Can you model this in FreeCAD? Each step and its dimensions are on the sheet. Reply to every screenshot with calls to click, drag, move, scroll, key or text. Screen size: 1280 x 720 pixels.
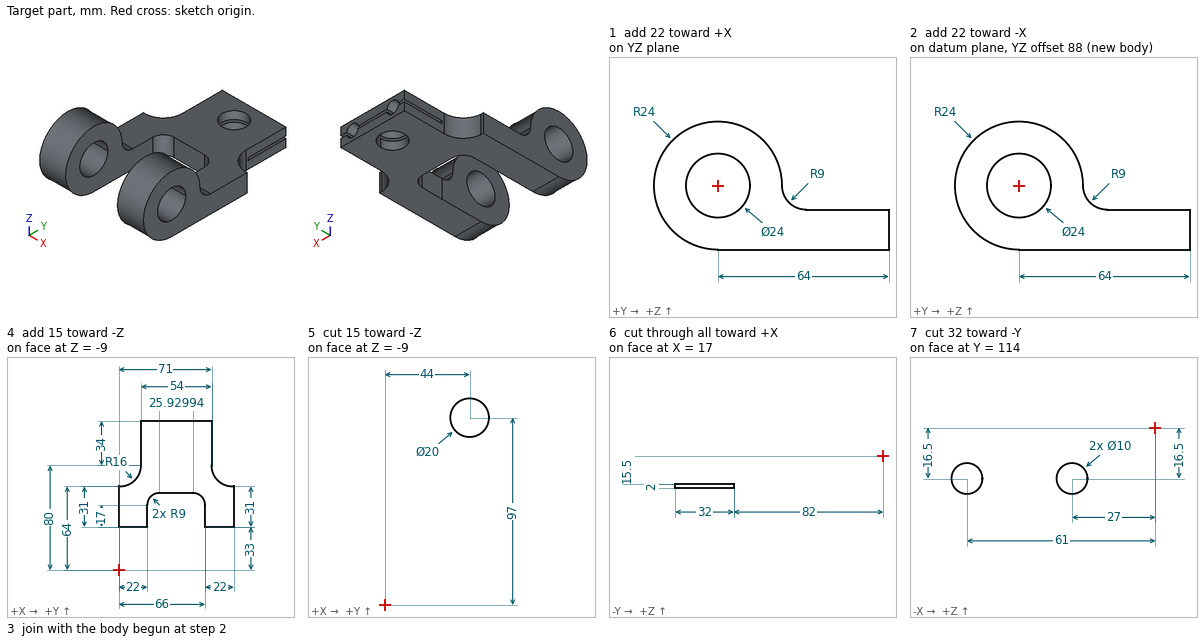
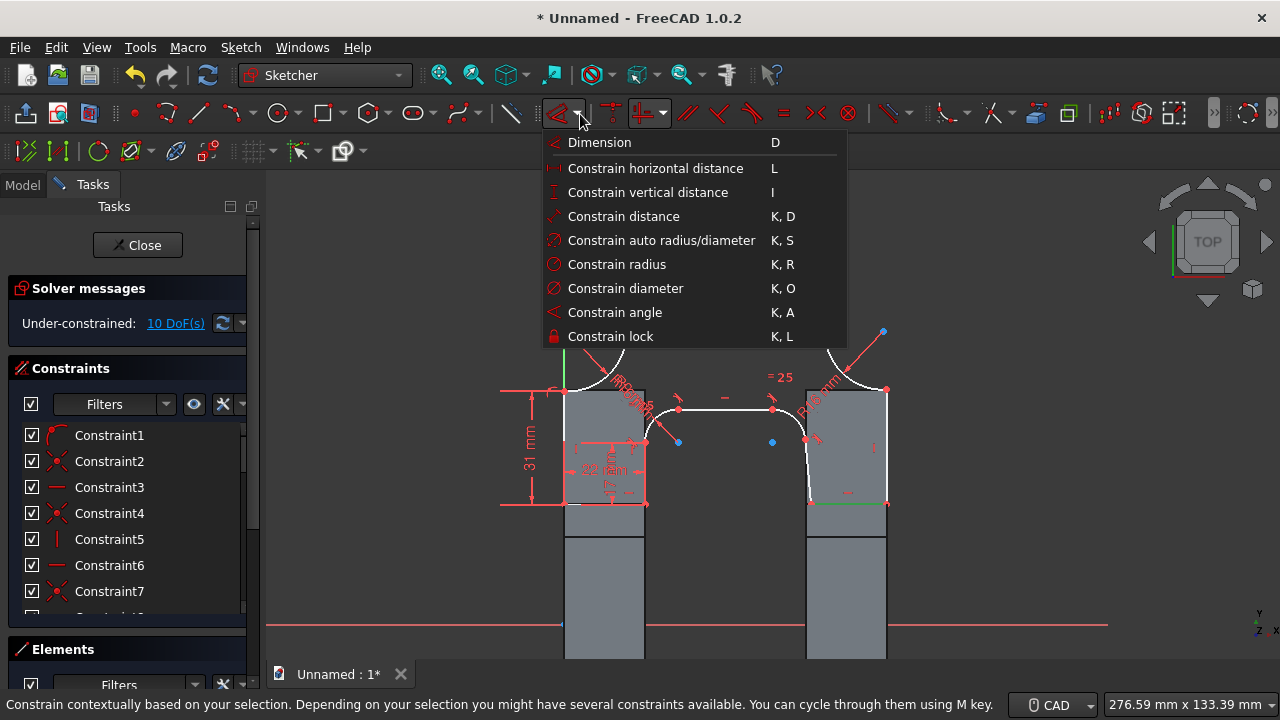
click(695, 168)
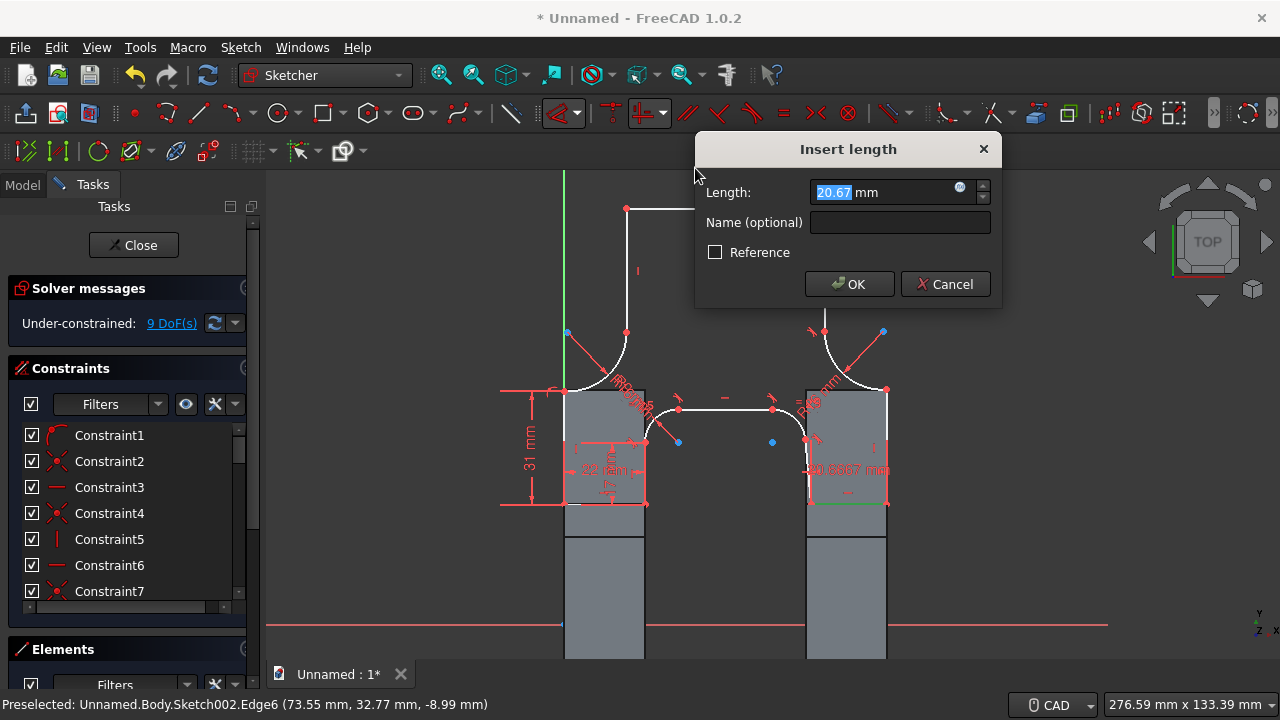
text(22)
key(Return)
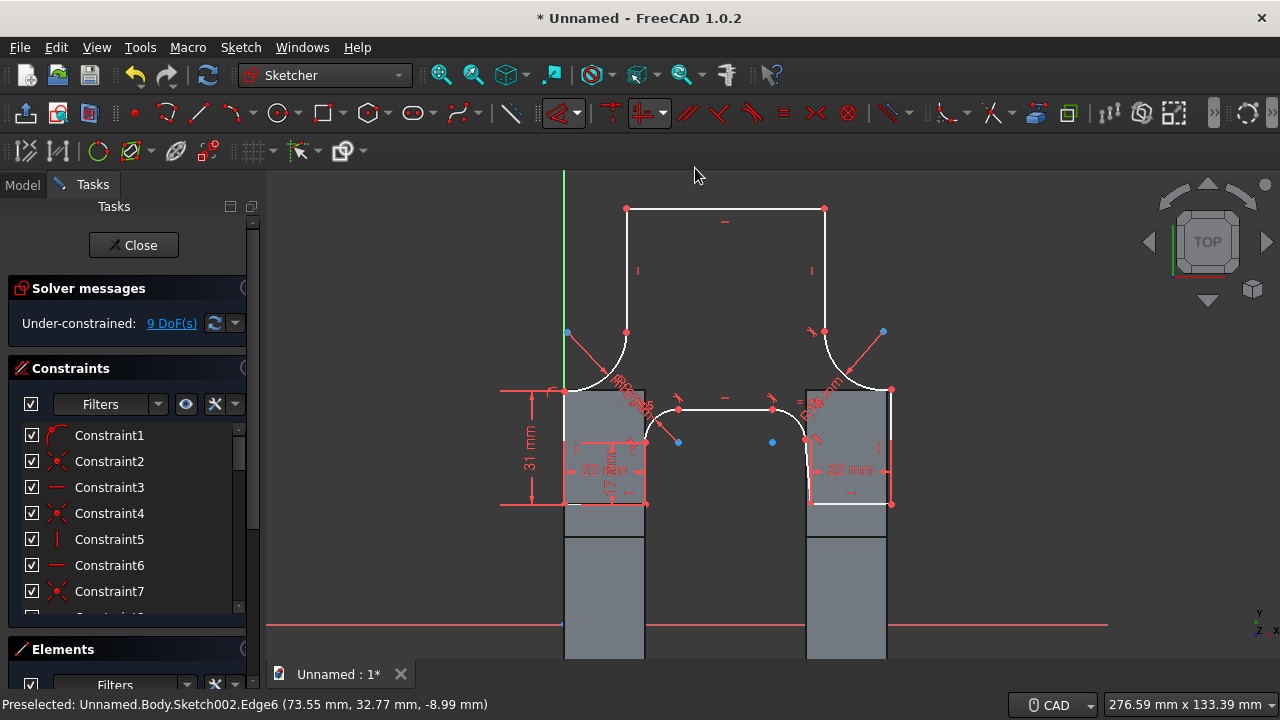
click(891, 470)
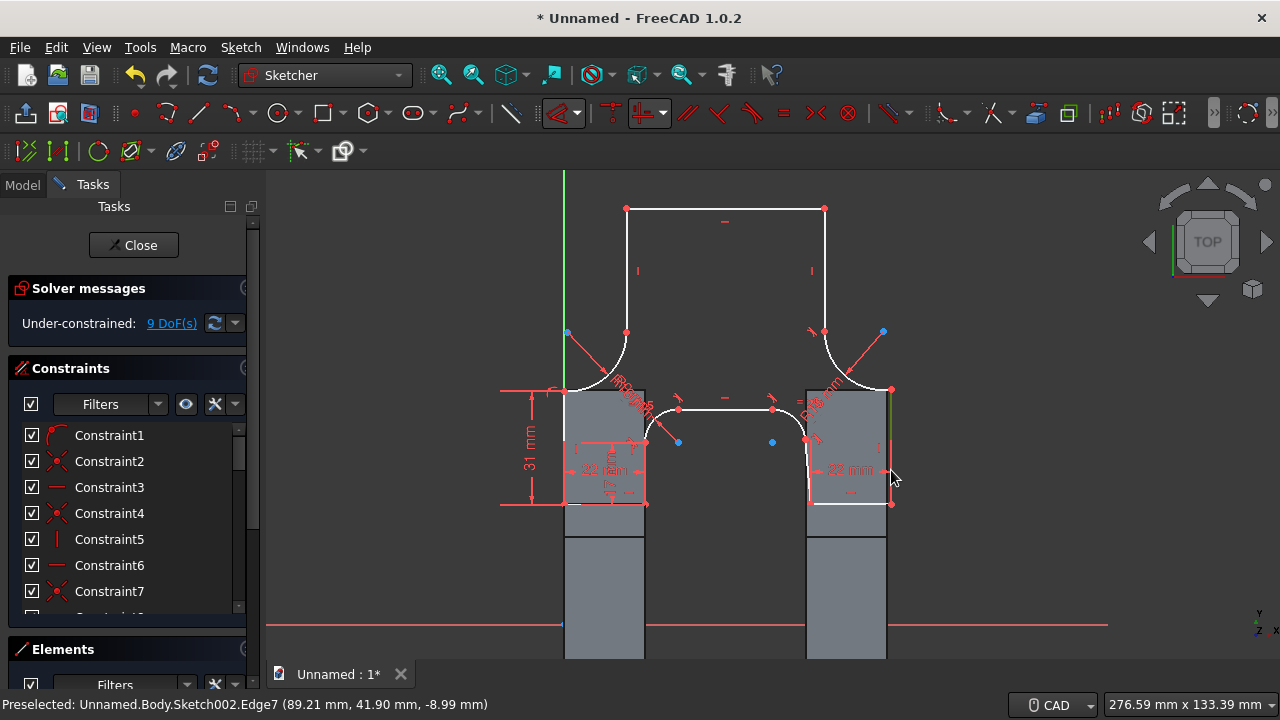
click(580, 114)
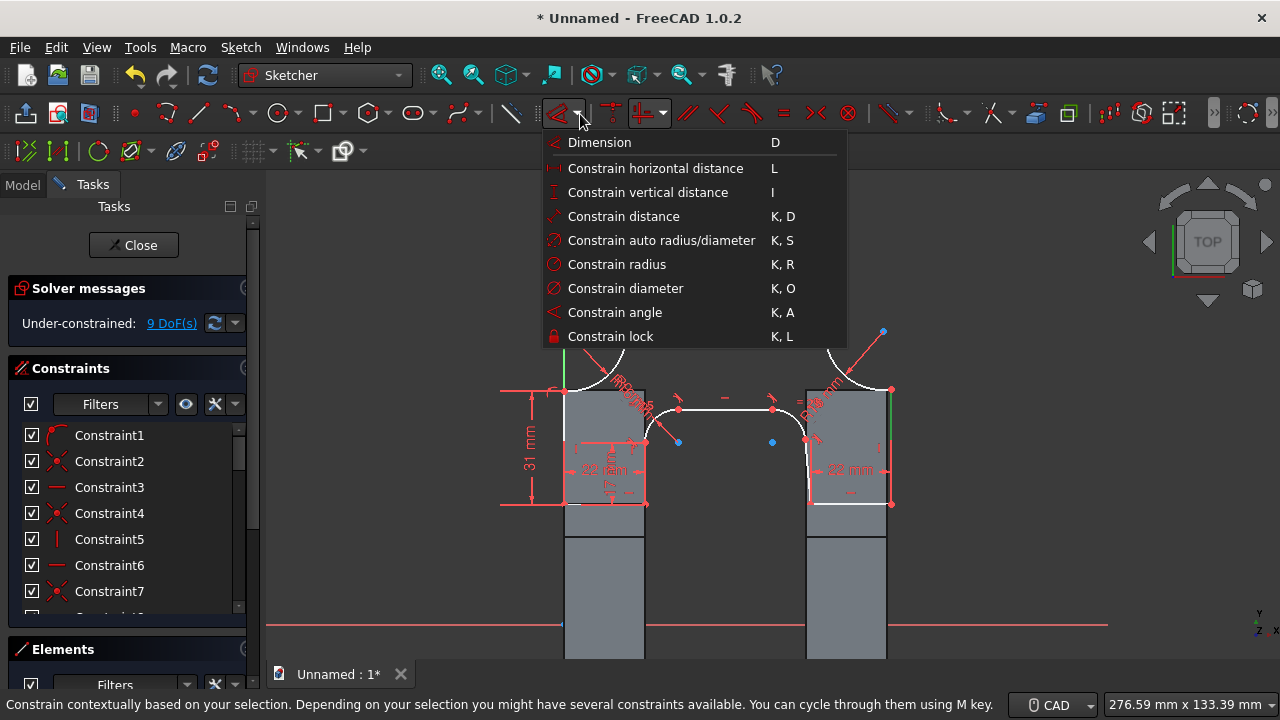
click(695, 192)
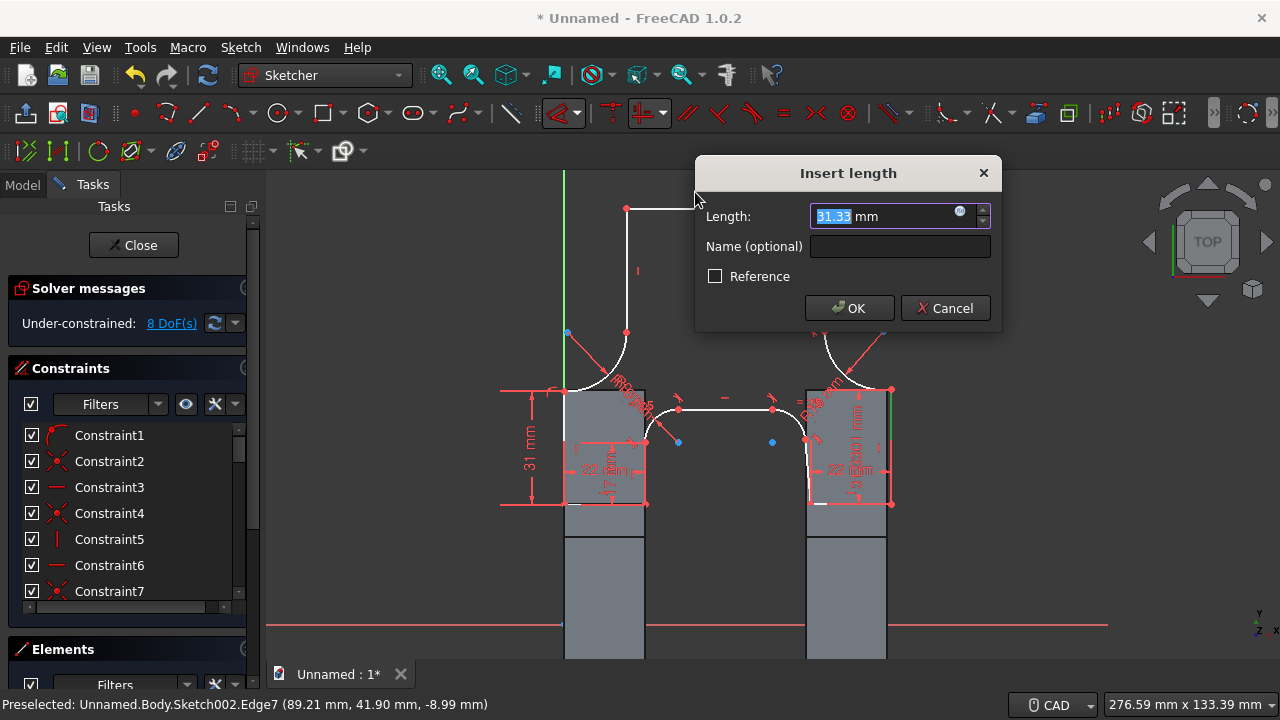
text(31)
key(Return)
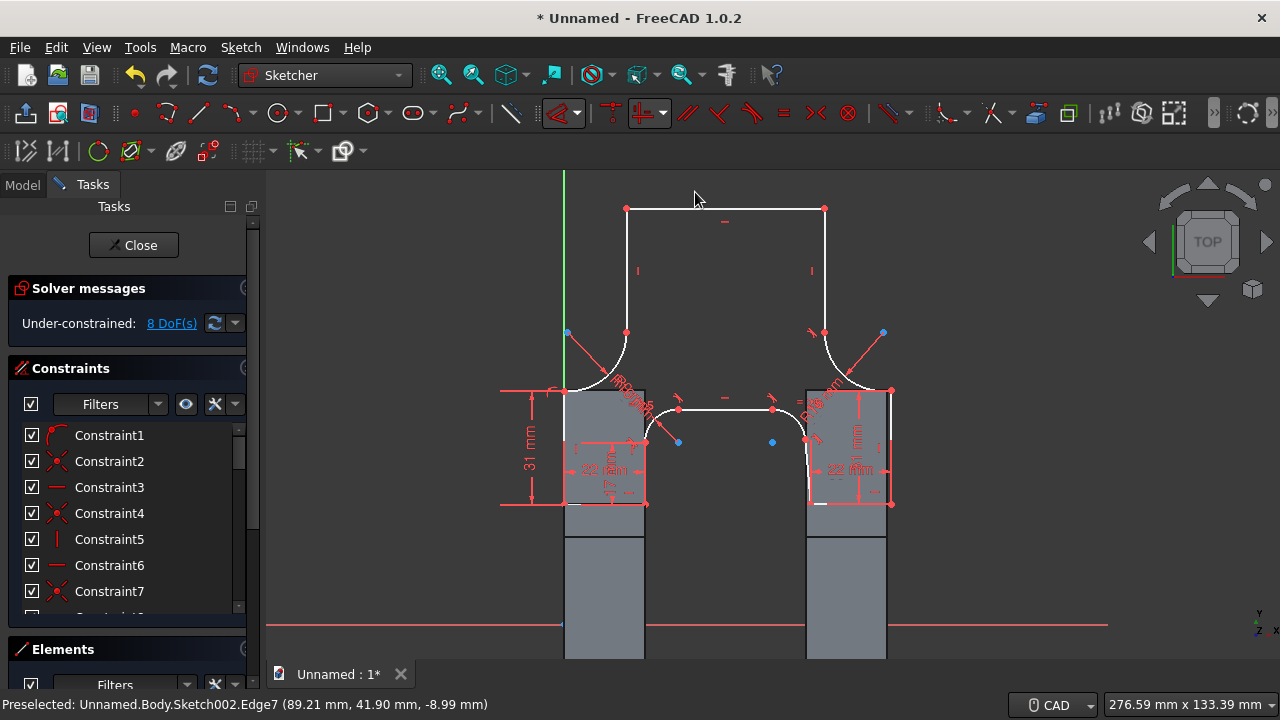
click(765, 209)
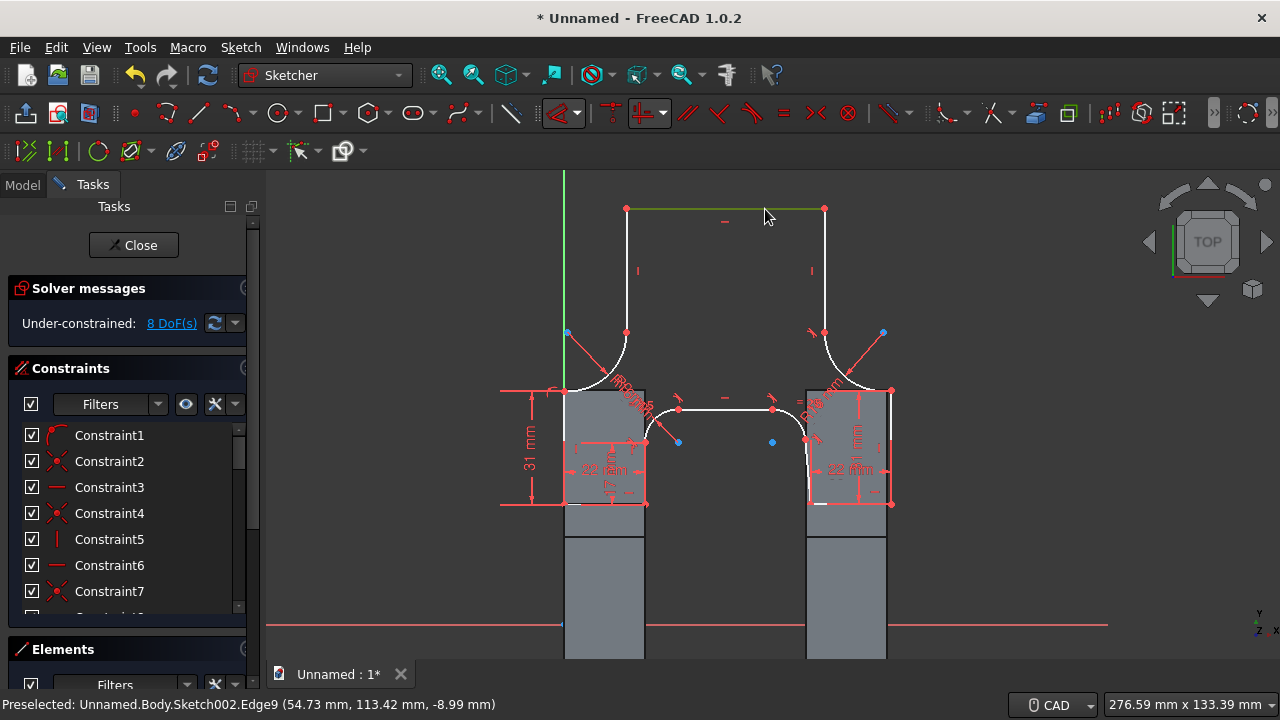
click(580, 114)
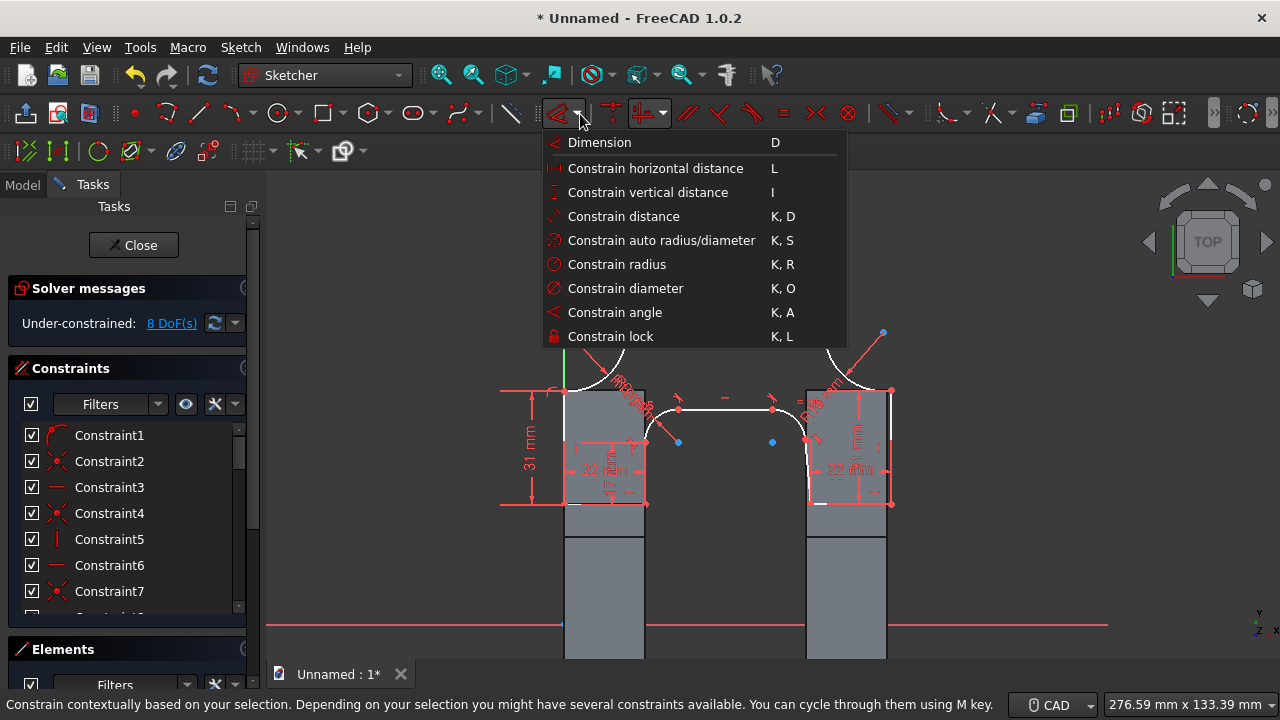
click(695, 168)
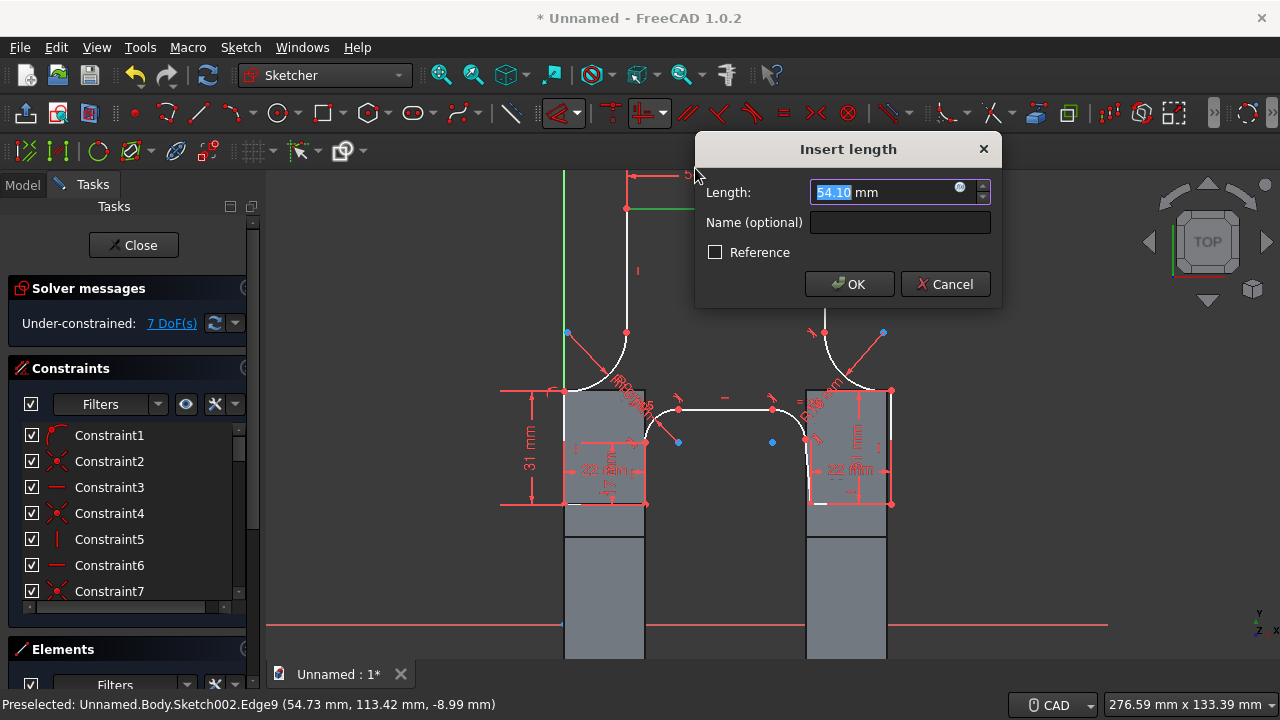
text(54)
key(Return)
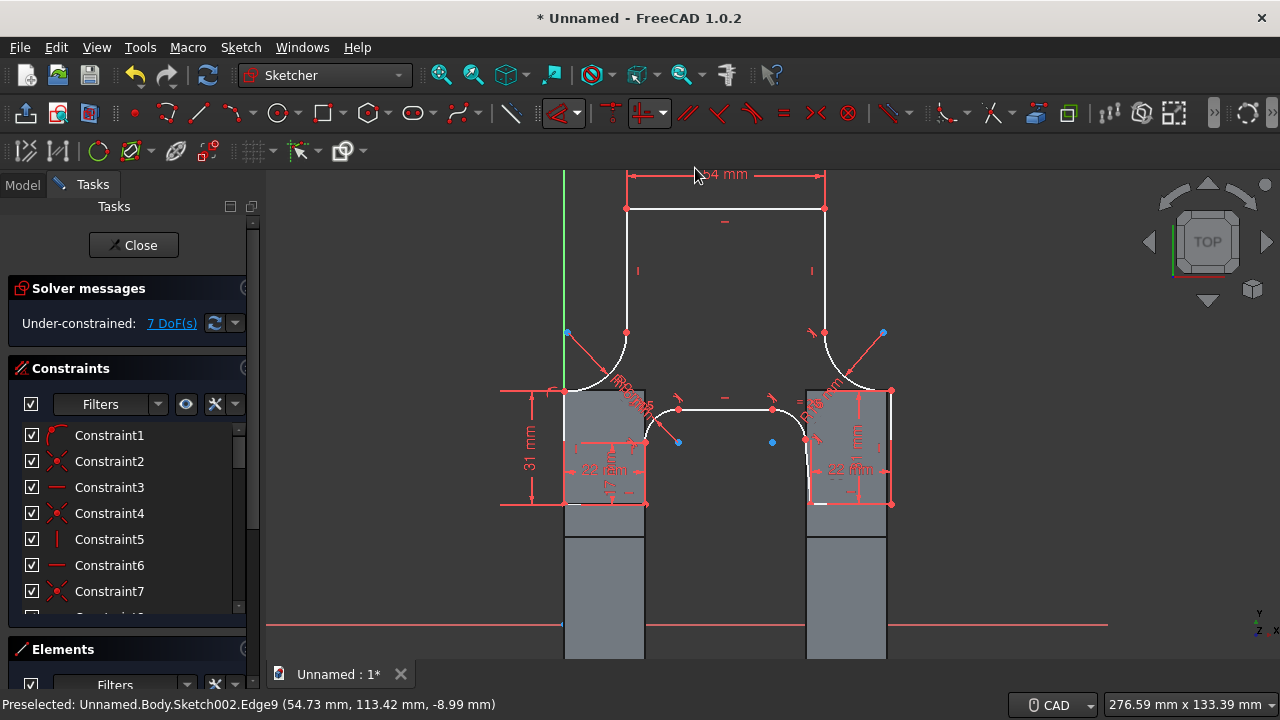
click(627, 246)